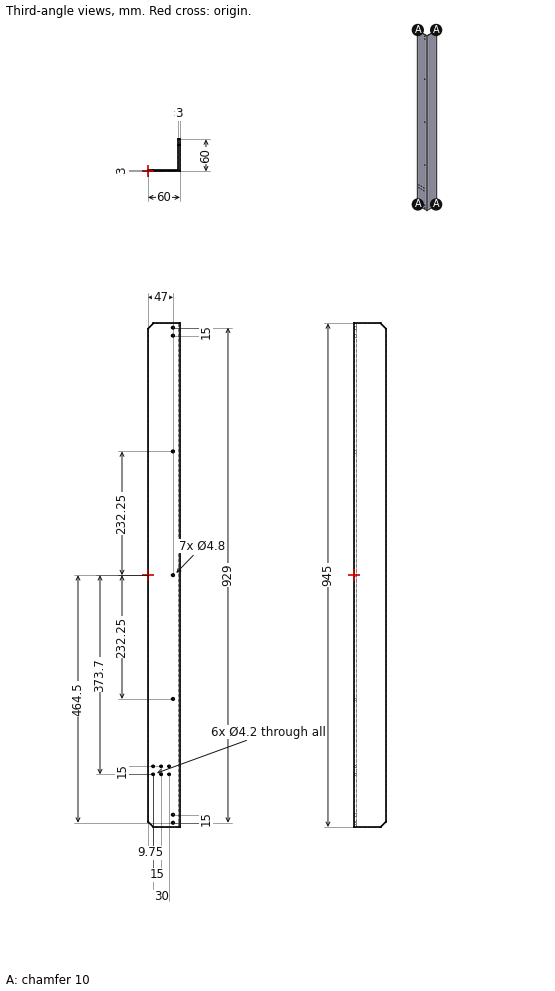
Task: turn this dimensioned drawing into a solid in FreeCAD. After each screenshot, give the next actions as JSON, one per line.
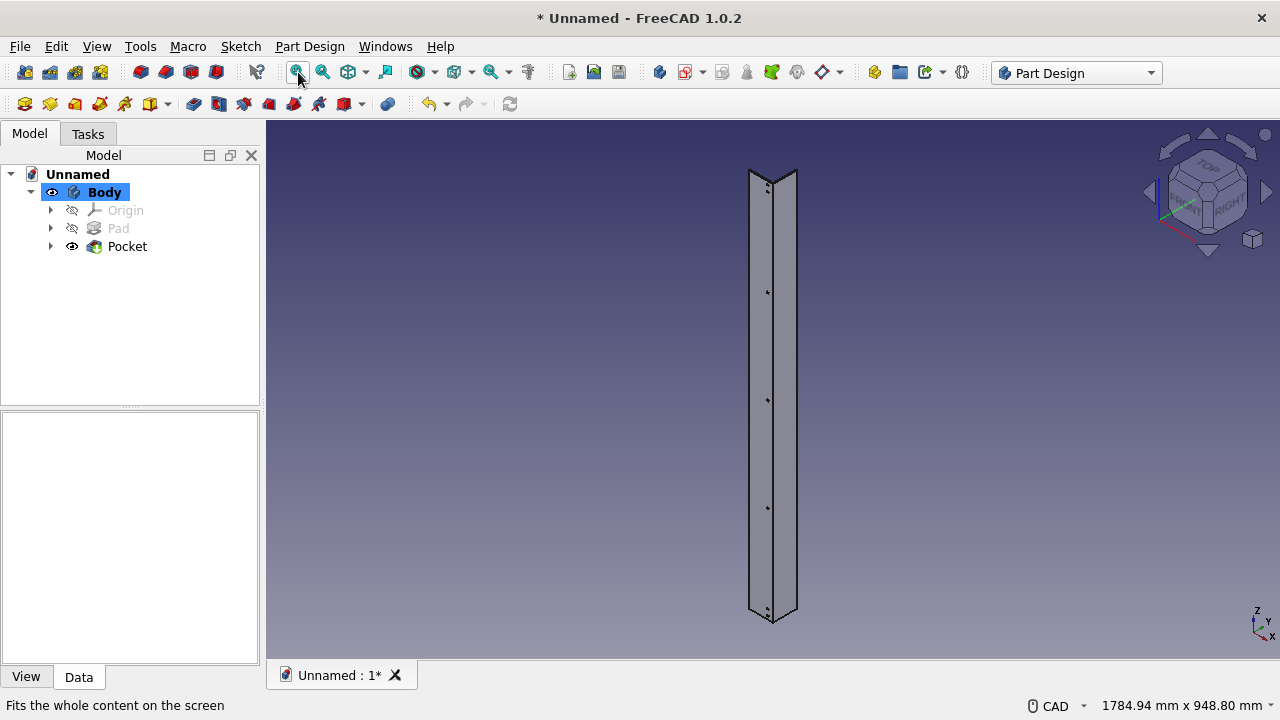
{"action": "key", "text": "2"}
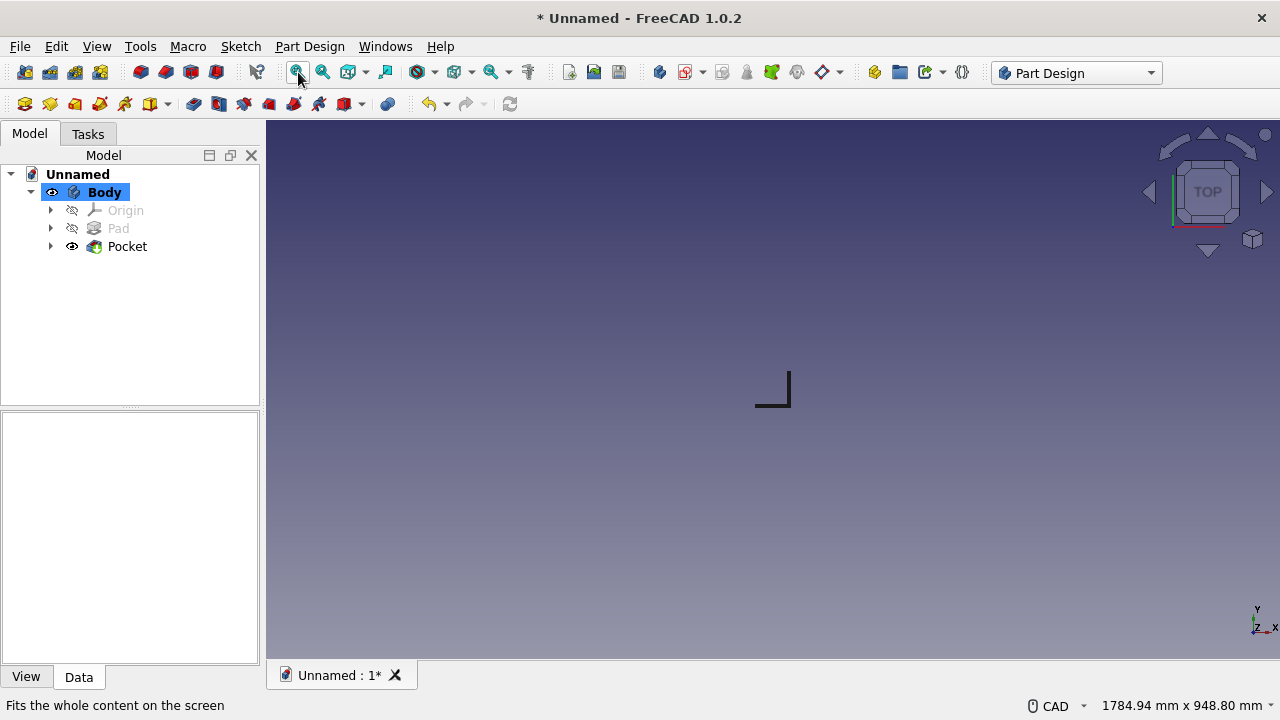
{"action": "left_click", "coordinate": [298, 72]}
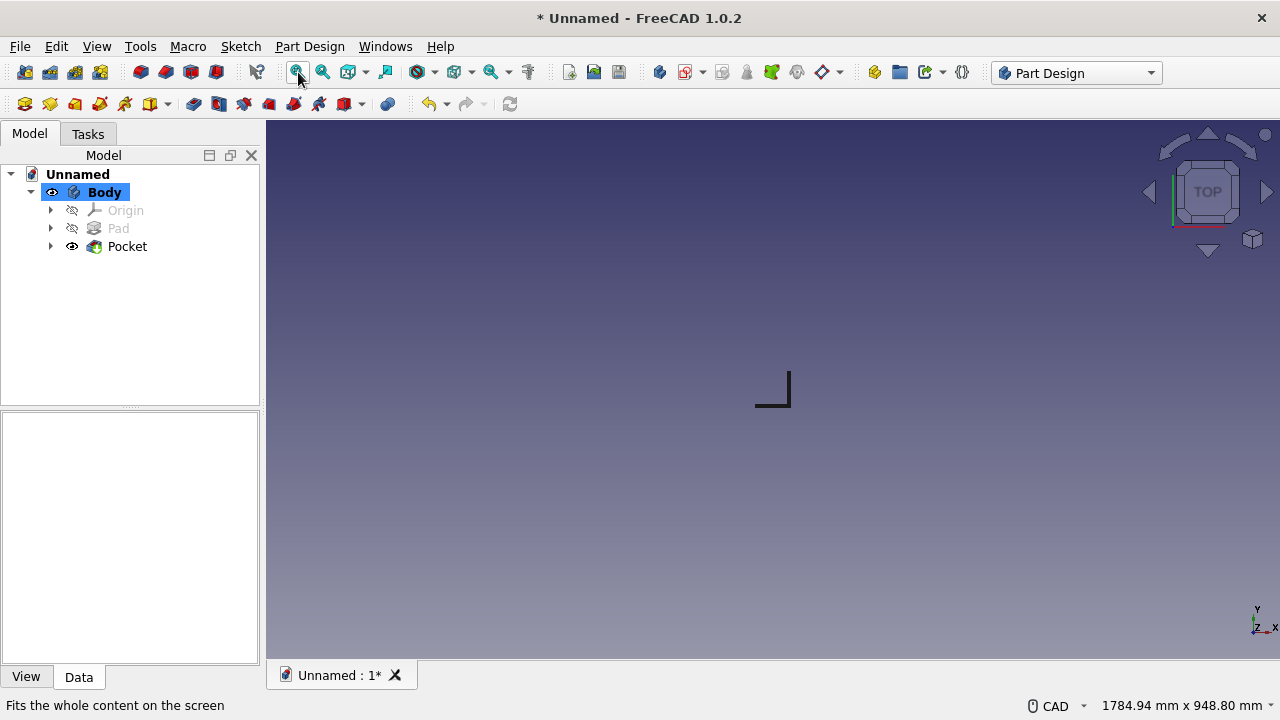
{"action": "scroll", "coordinate": [789, 371], "scroll_direction": "up", "scroll_amount": 15}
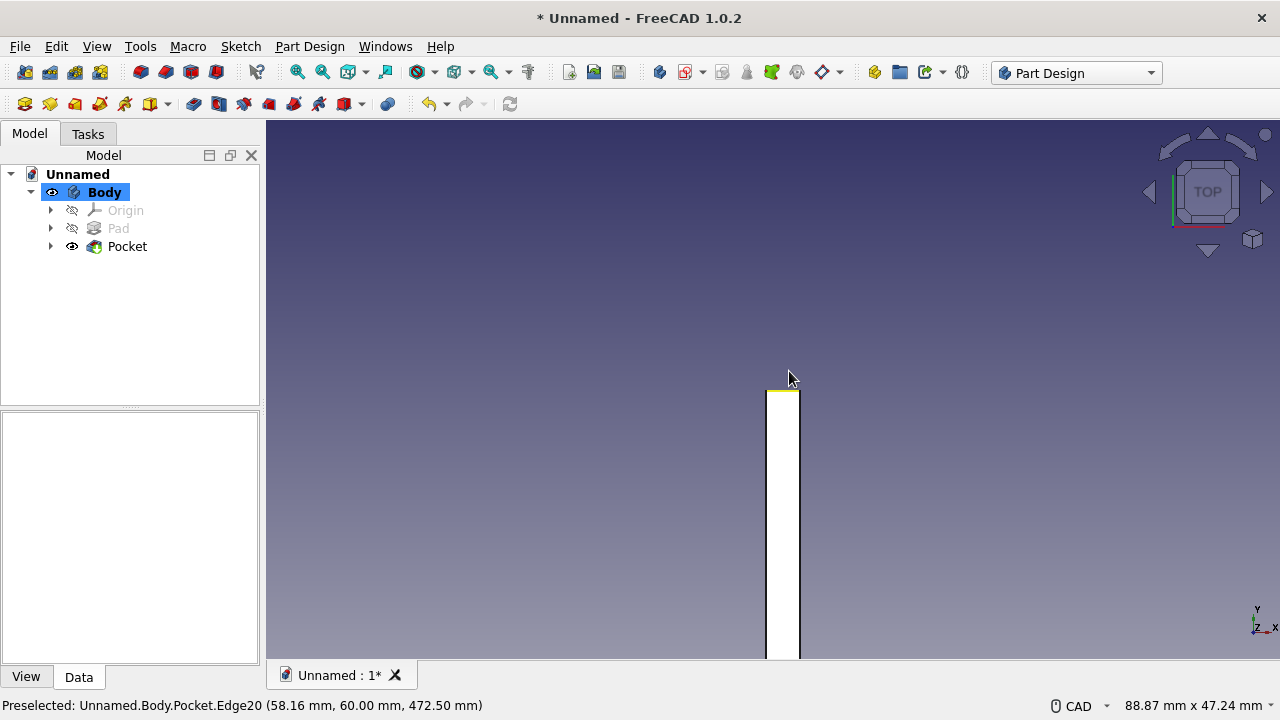
{"action": "left_click", "coordinate": [783, 390]}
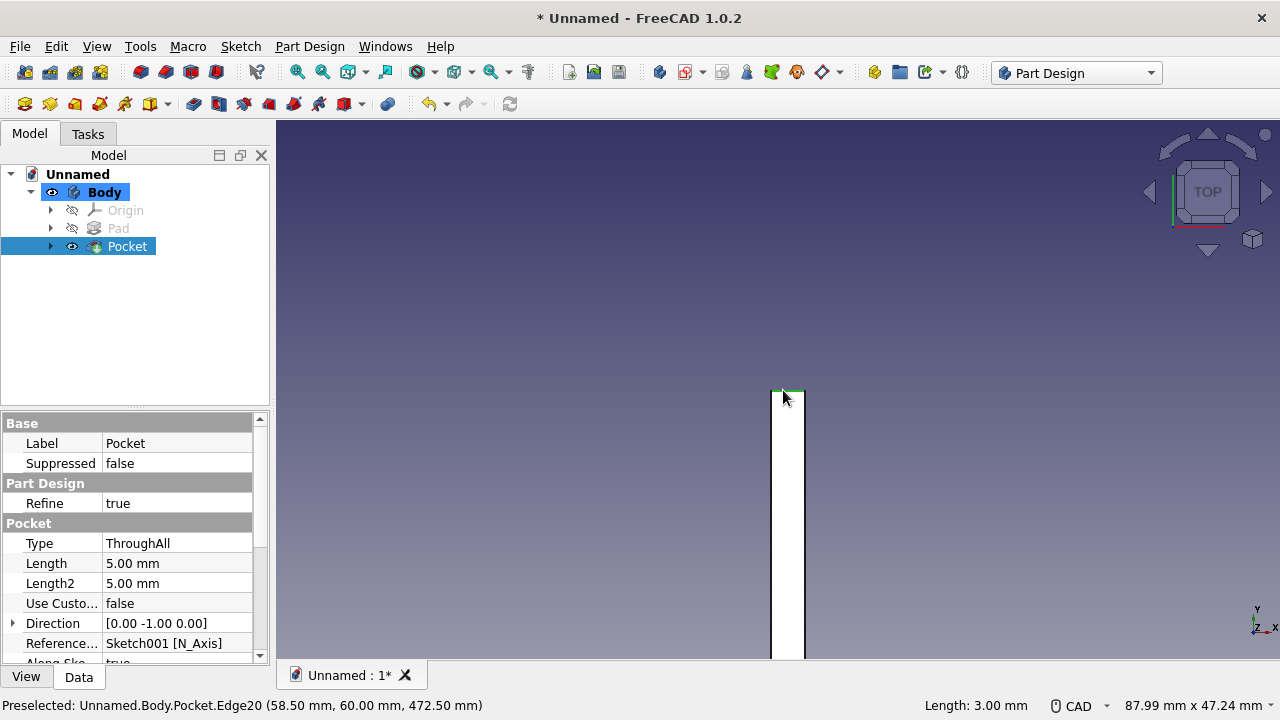
{"action": "left_click", "coordinate": [298, 72]}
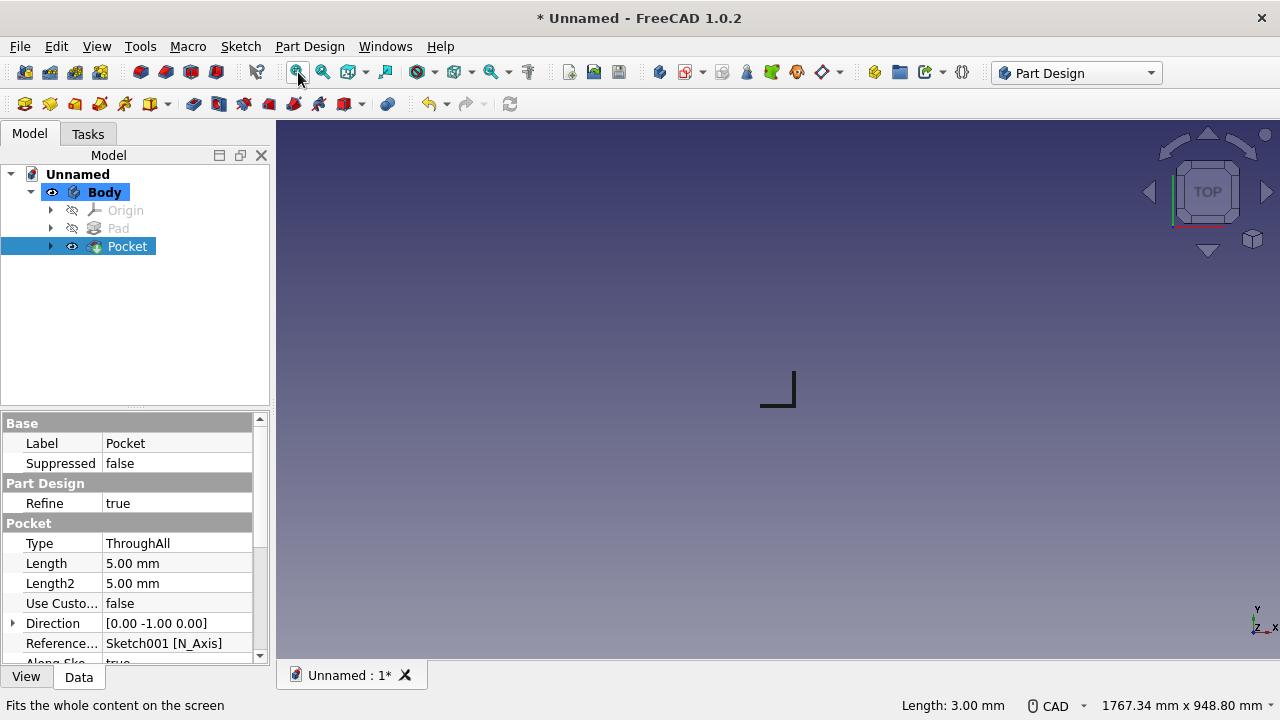
{"action": "key", "text": "1"}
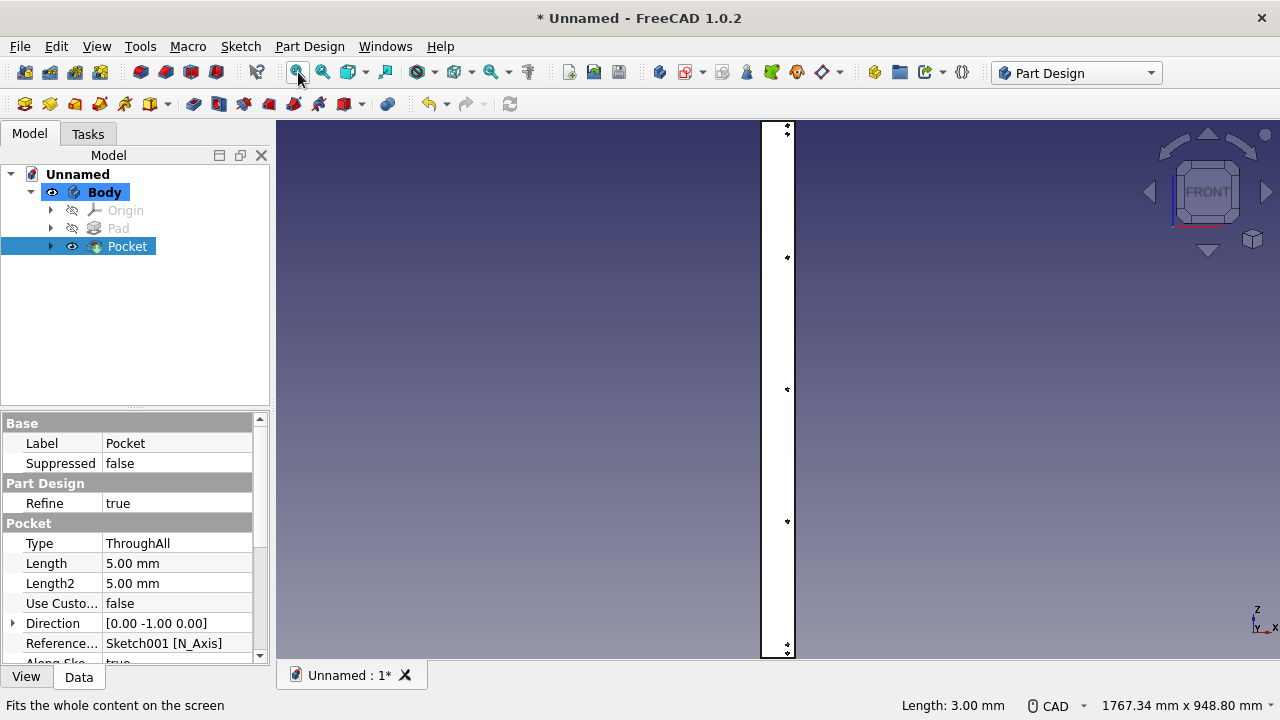
{"action": "key", "text": "3"}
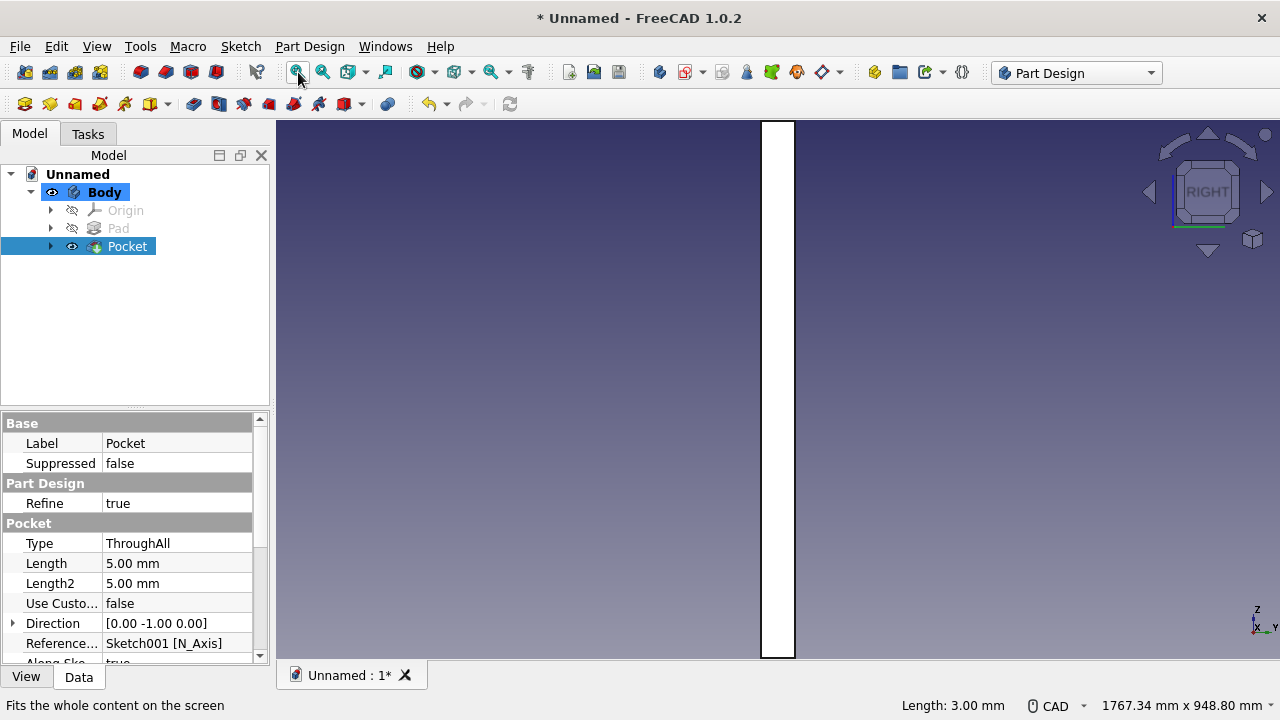
{"action": "key", "text": "5"}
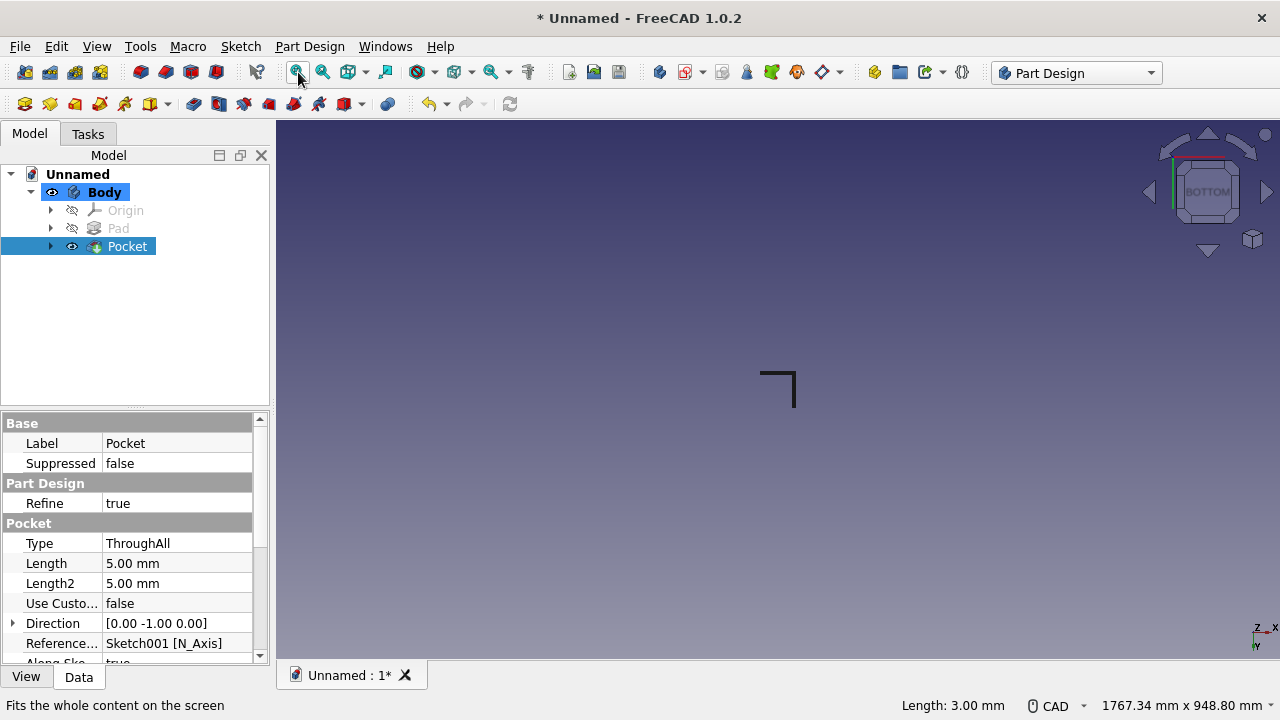
{"action": "left_click", "coordinate": [298, 72]}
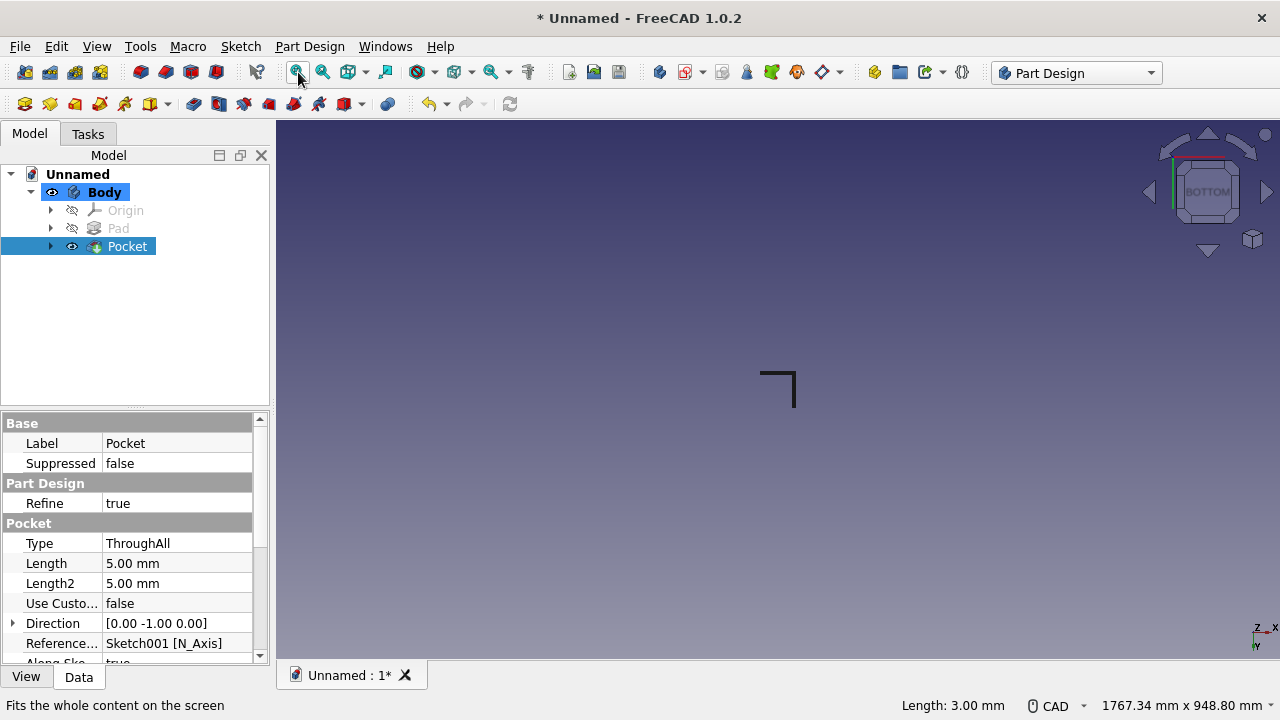
{"action": "scroll", "coordinate": [761, 372], "scroll_direction": "up", "scroll_amount": 15}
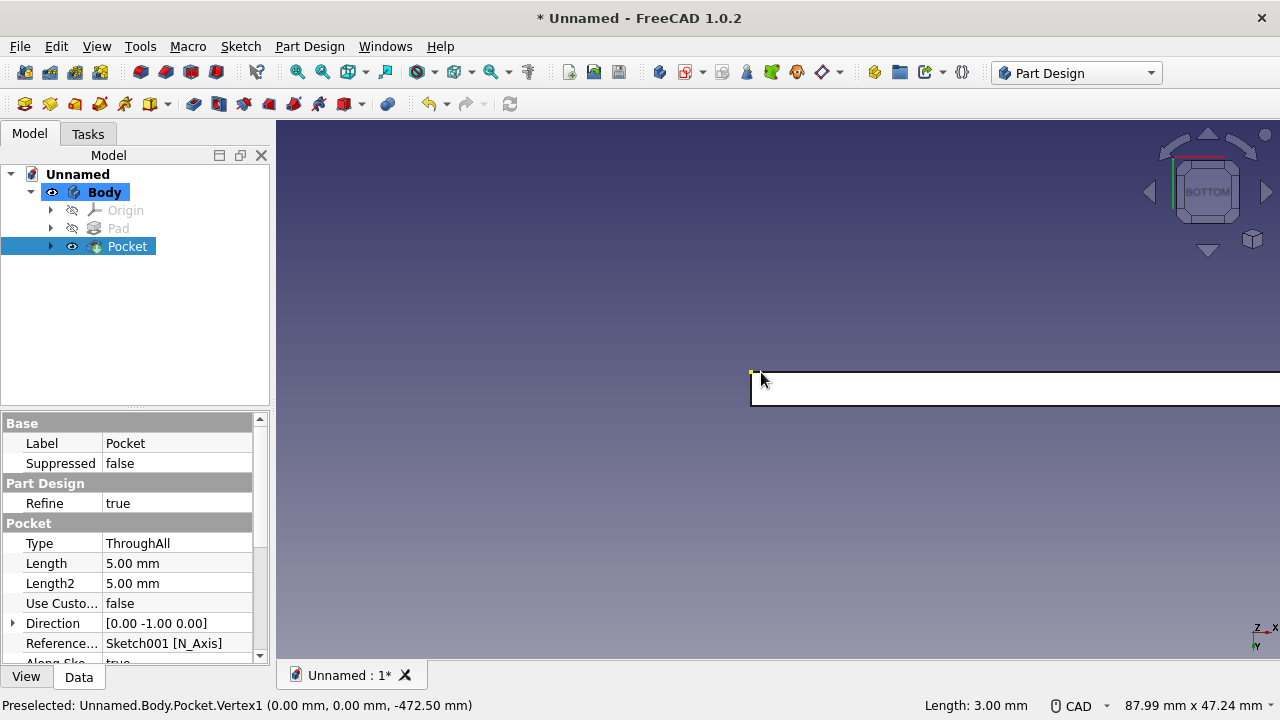
{"action": "left_click", "coordinate": [751, 388], "text": "ctrl"}